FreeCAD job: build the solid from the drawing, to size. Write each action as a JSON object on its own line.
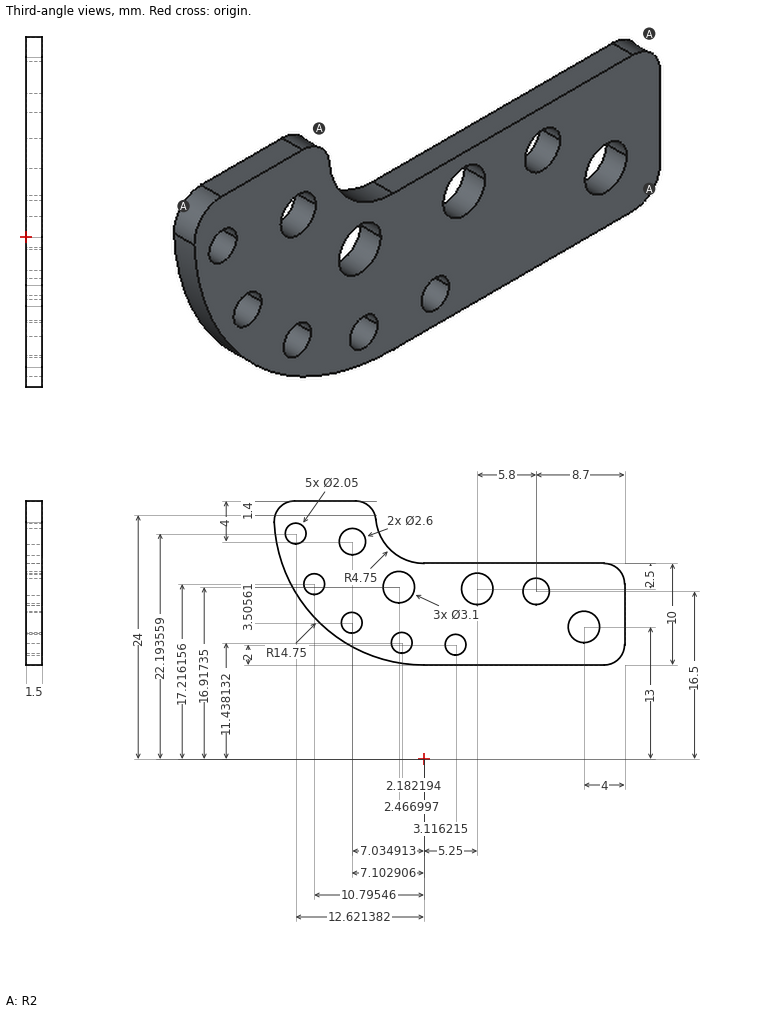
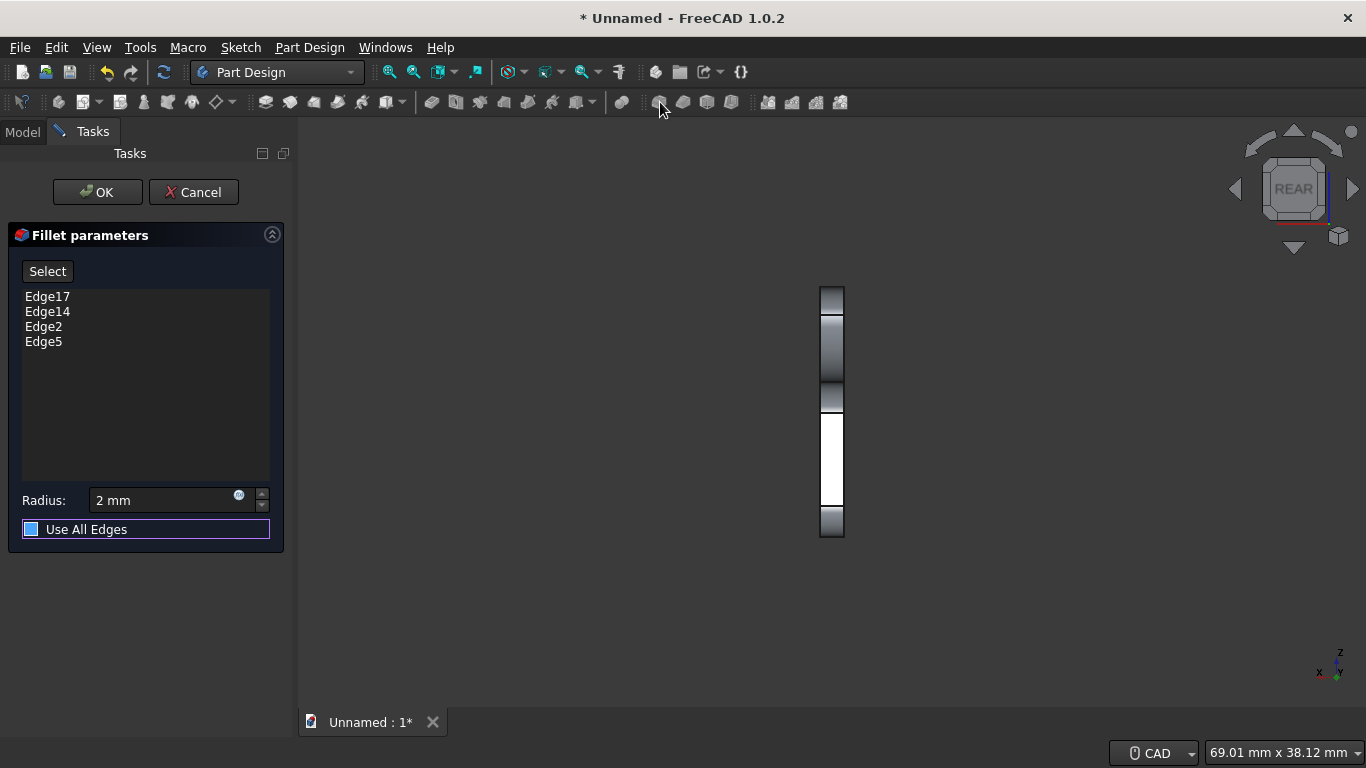
{"action": "left_click", "coordinate": [98, 192]}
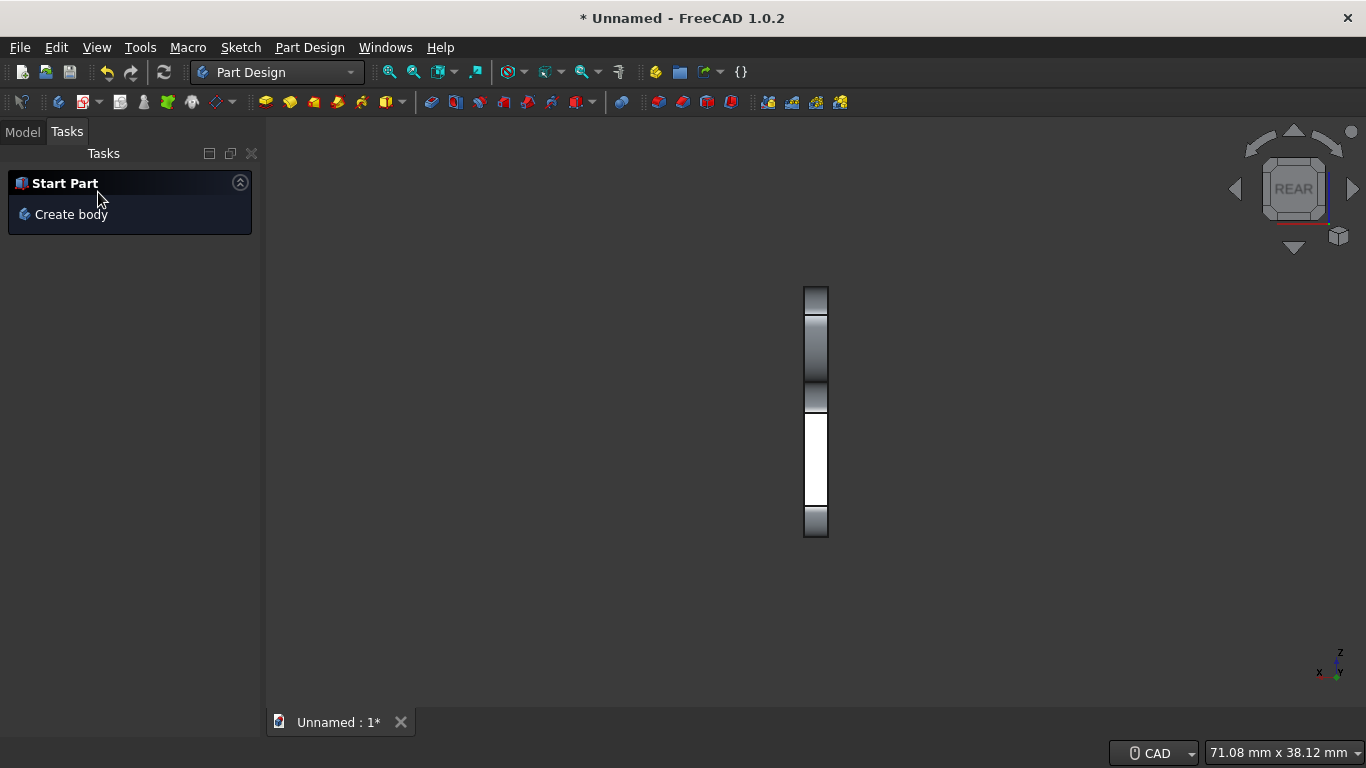
{"action": "key", "text": "0"}